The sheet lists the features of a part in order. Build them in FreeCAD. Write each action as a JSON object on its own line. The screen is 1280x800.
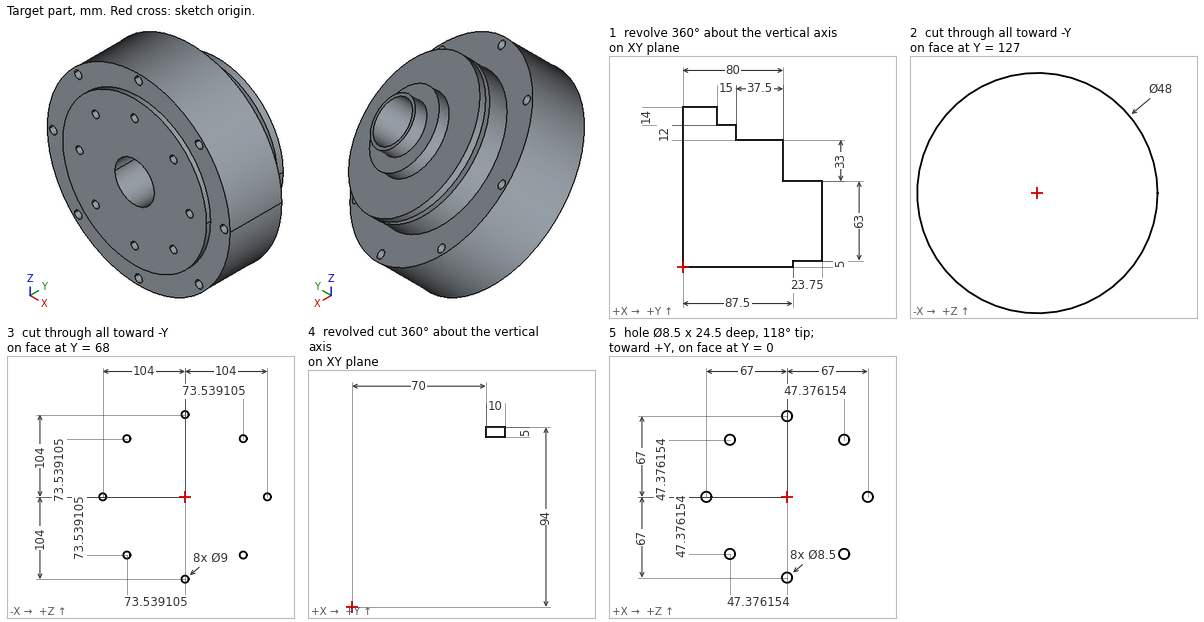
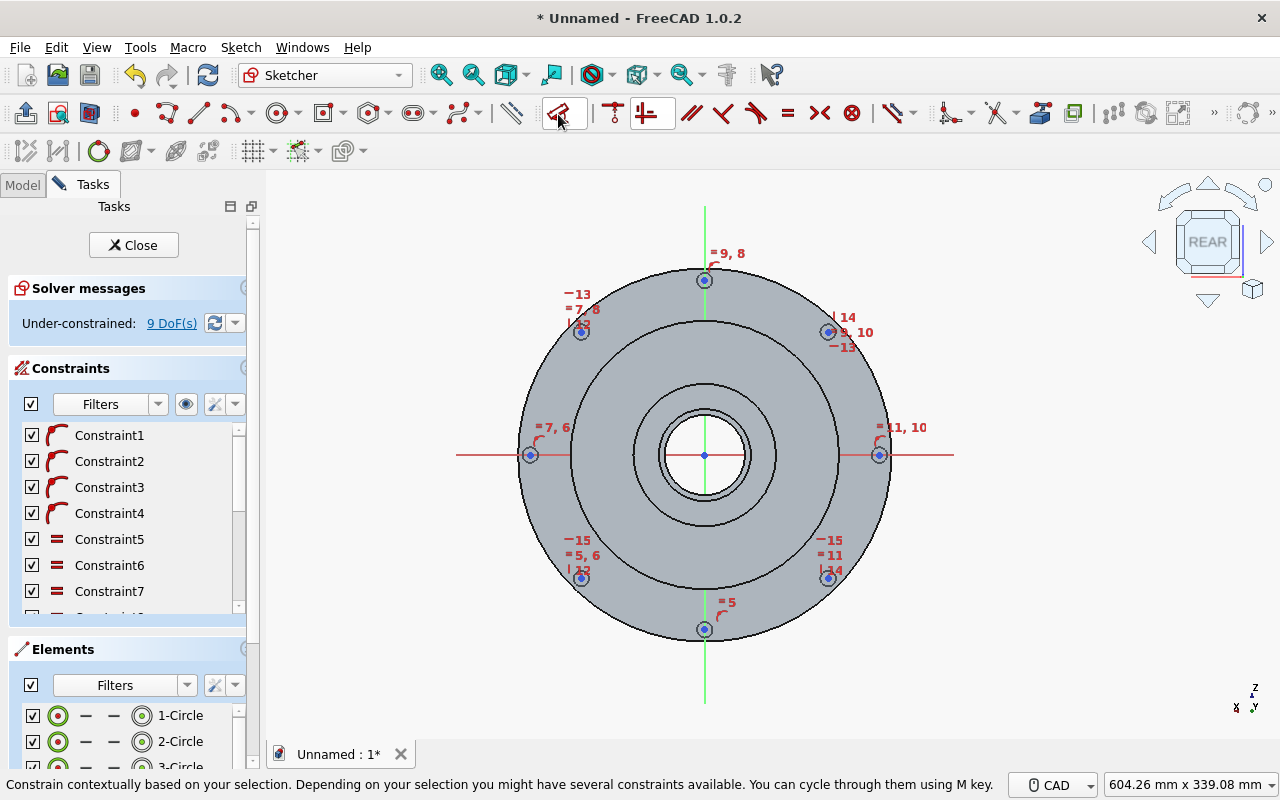
{"action": "scroll", "coordinate": [705, 622], "scroll_direction": "up", "scroll_amount": 5}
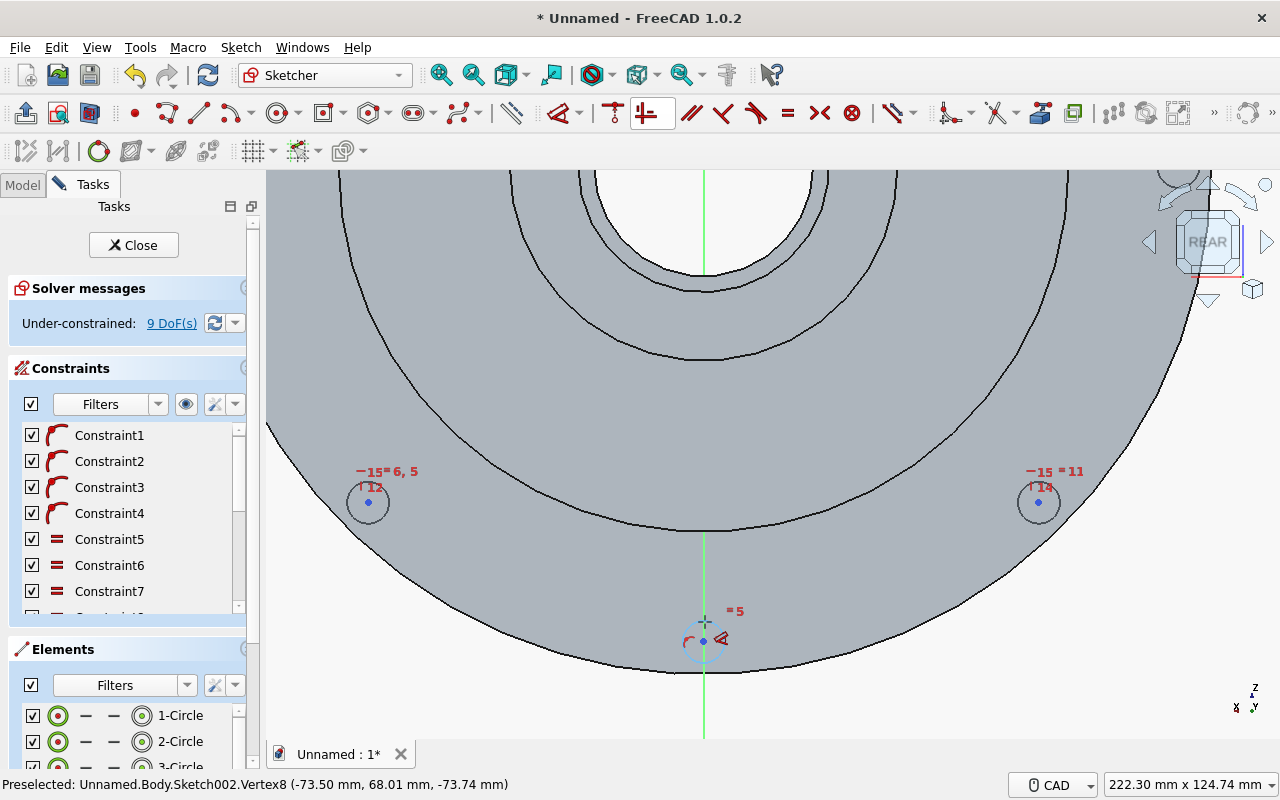
{"action": "left_click", "coordinate": [704, 621]}
{"action": "left_click", "coordinate": [730, 596]}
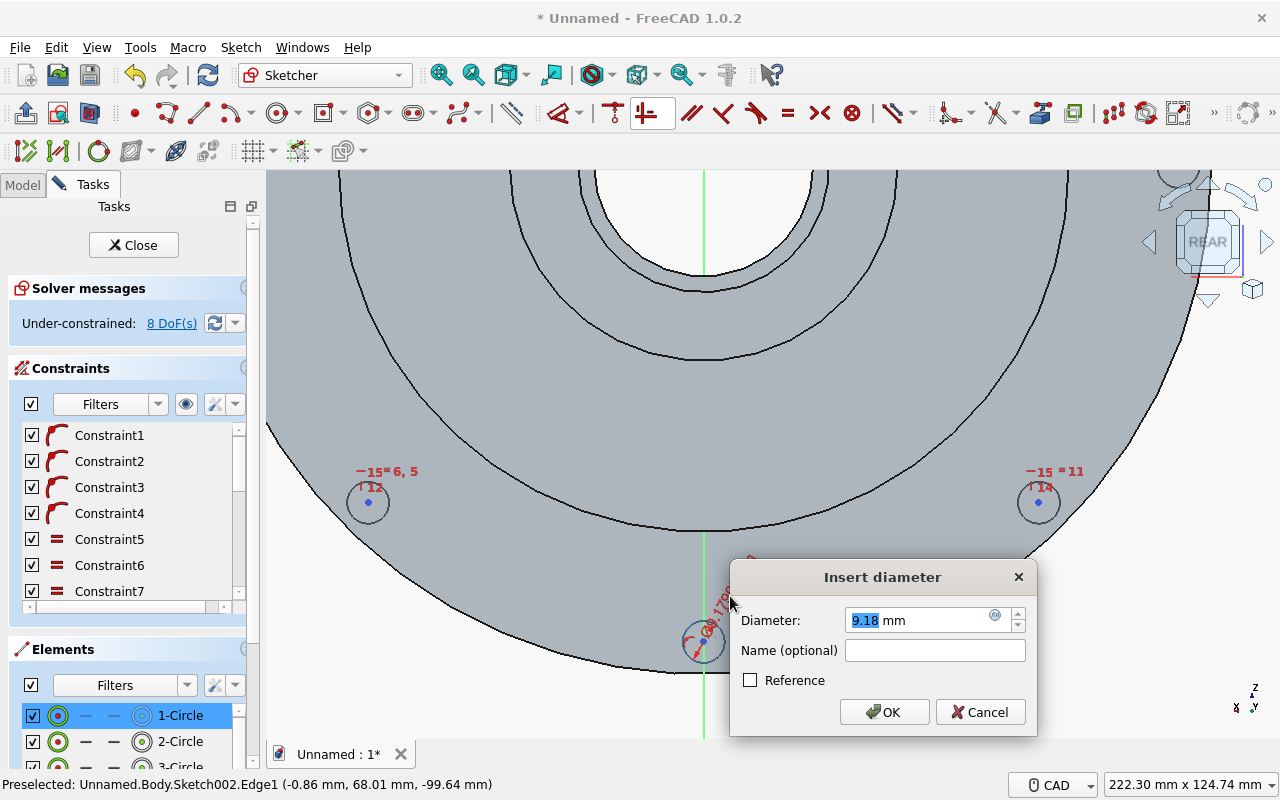
{"action": "type", "text": "9"}
{"action": "key", "text": "Return"}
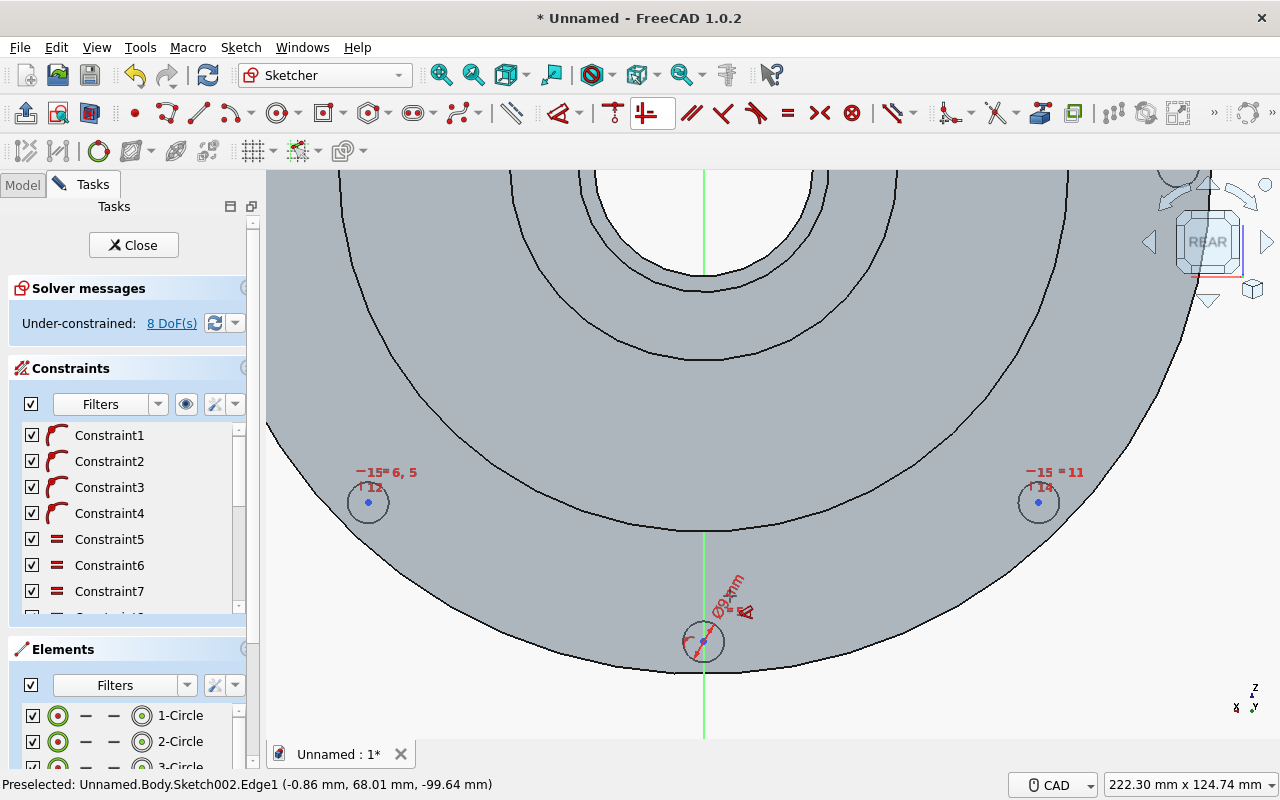
{"action": "left_click", "coordinate": [704, 642]}
{"action": "left_click", "coordinate": [738, 420]}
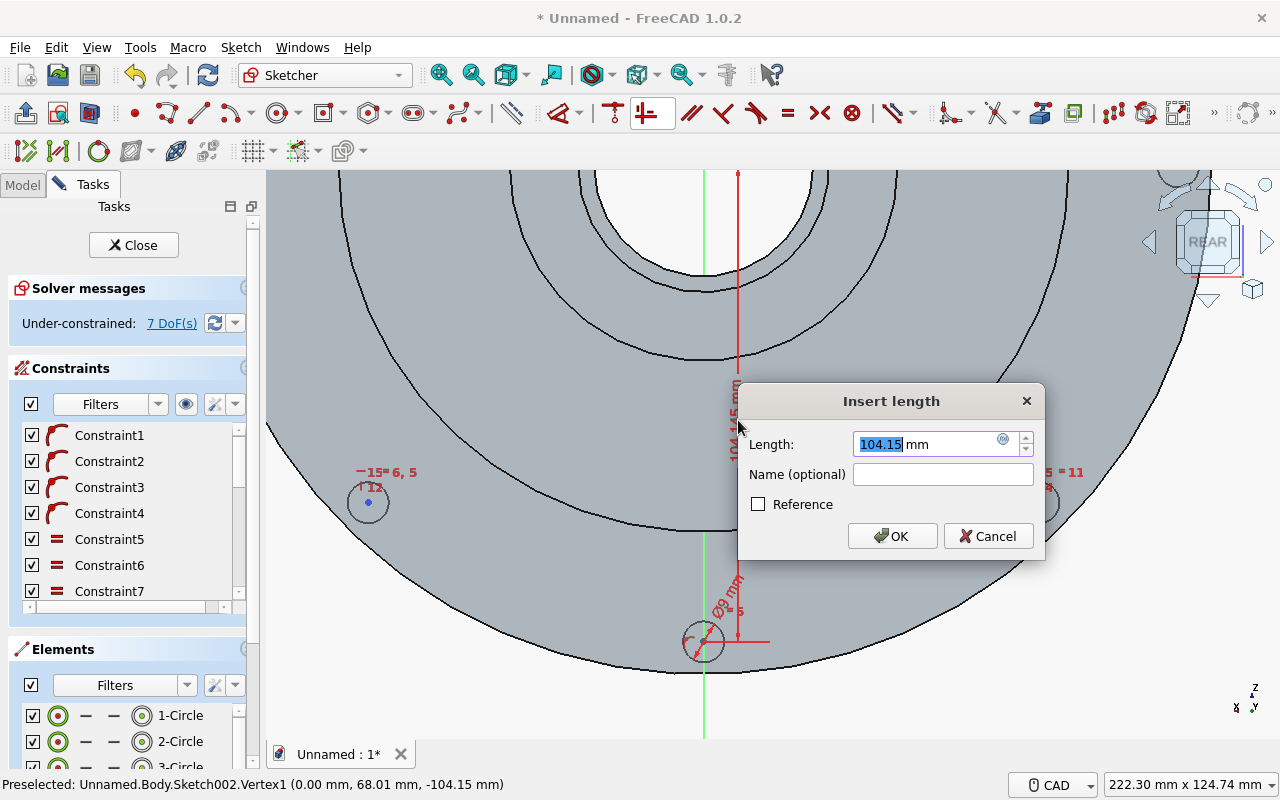
{"action": "type", "text": "104"}
{"action": "key", "text": "Return"}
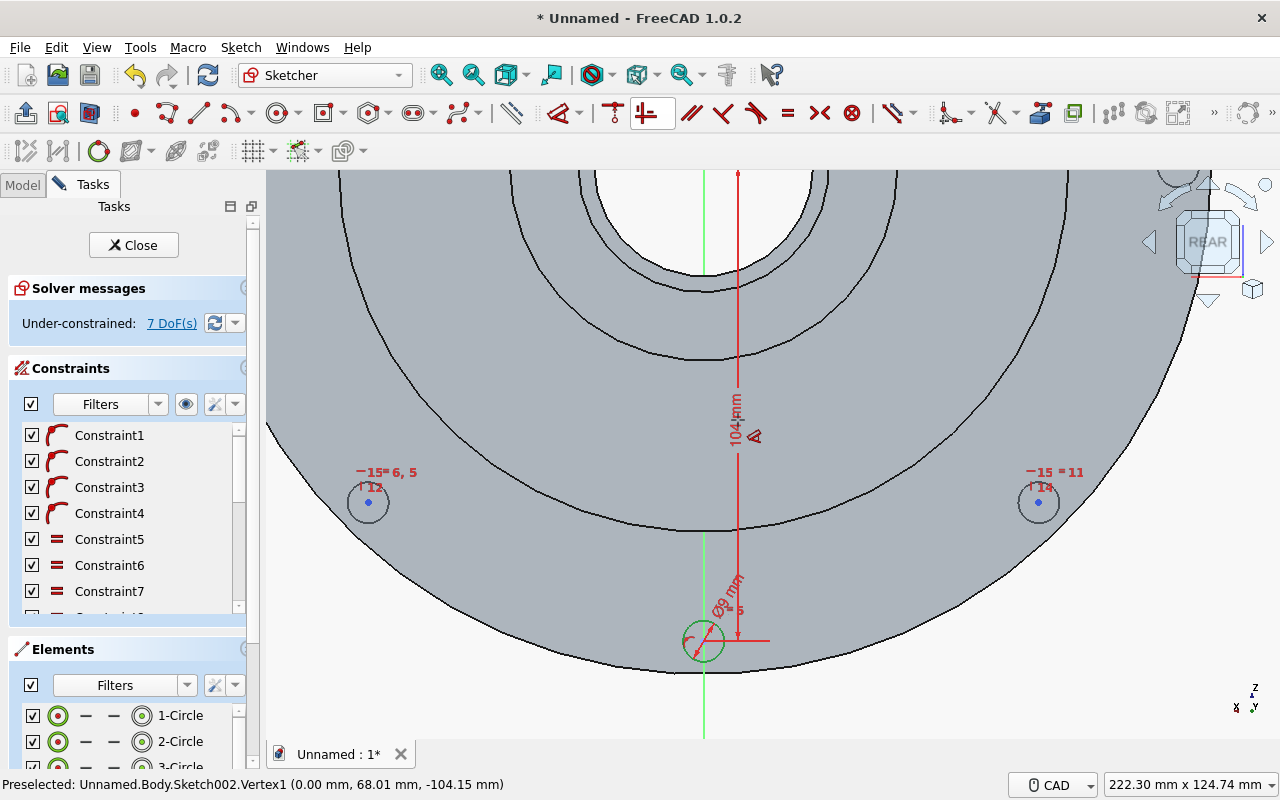
{"action": "scroll", "coordinate": [705, 622], "scroll_direction": "down", "scroll_amount": 5}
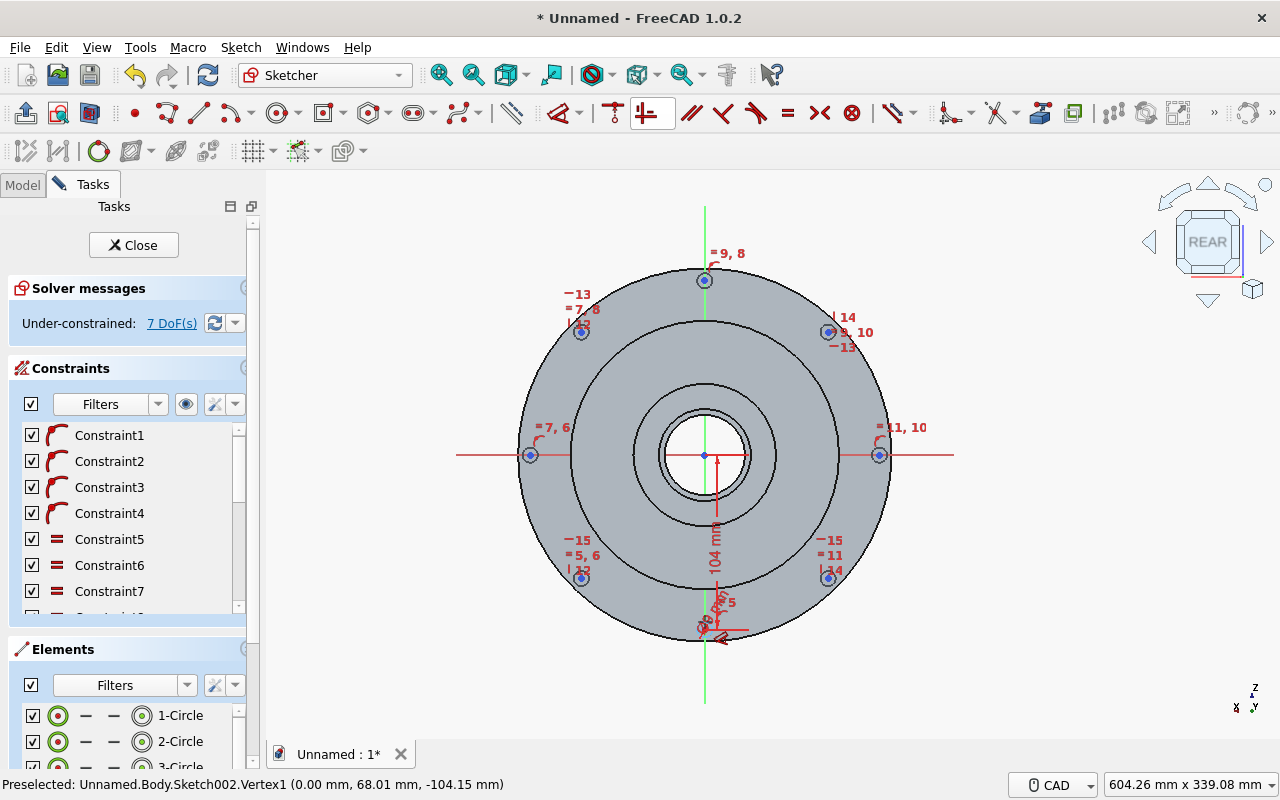
{"action": "left_click", "coordinate": [530, 455]}
{"action": "left_click", "coordinate": [618, 489]}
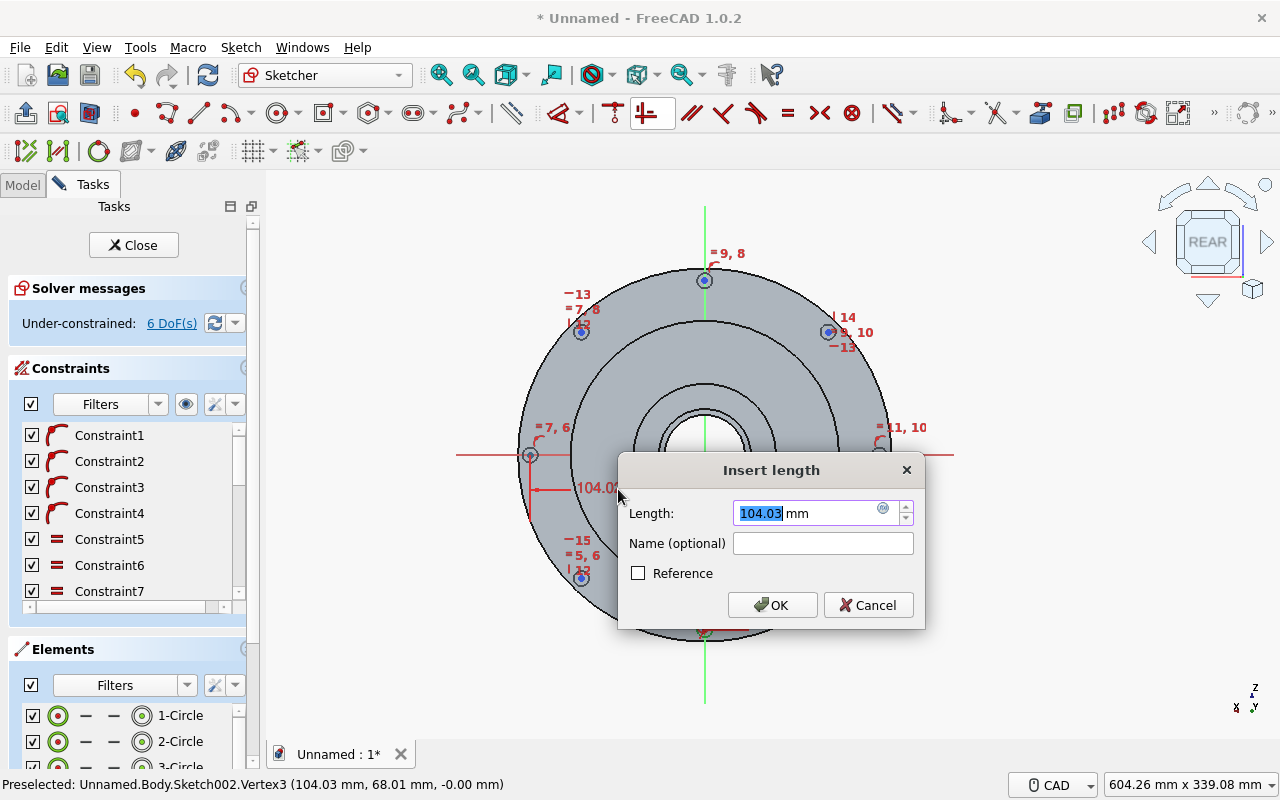
{"action": "type", "text": "104"}
{"action": "key", "text": "Return"}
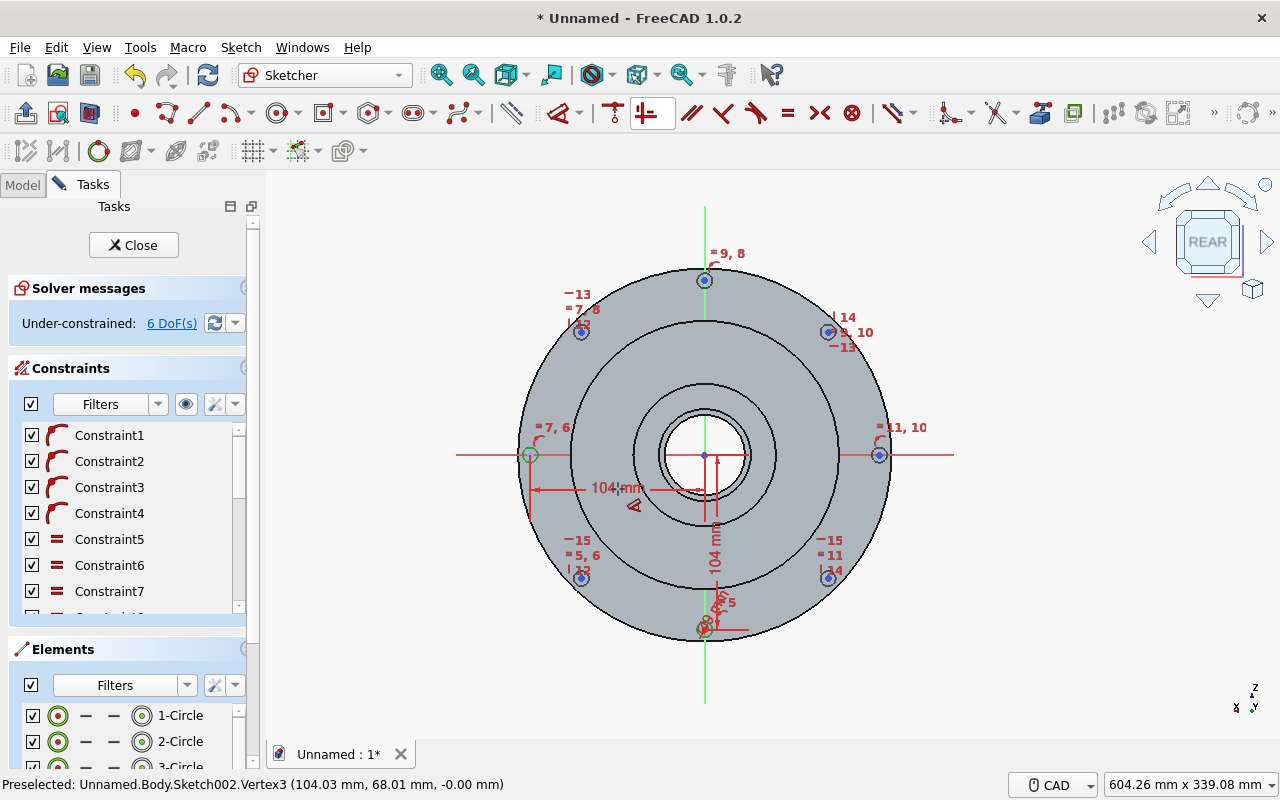
{"action": "left_click", "coordinate": [705, 281]}
{"action": "left_click", "coordinate": [739, 368]}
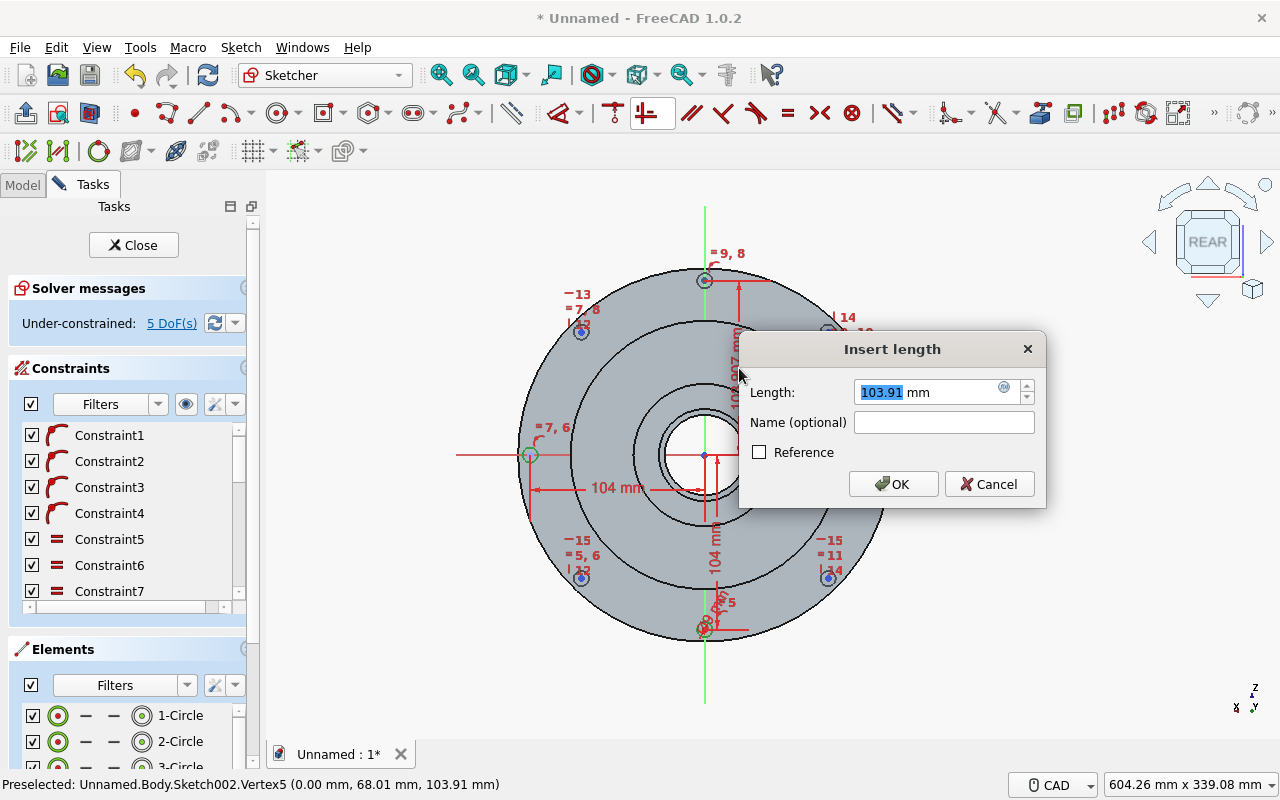
{"action": "type", "text": "104"}
{"action": "key", "text": "Return"}